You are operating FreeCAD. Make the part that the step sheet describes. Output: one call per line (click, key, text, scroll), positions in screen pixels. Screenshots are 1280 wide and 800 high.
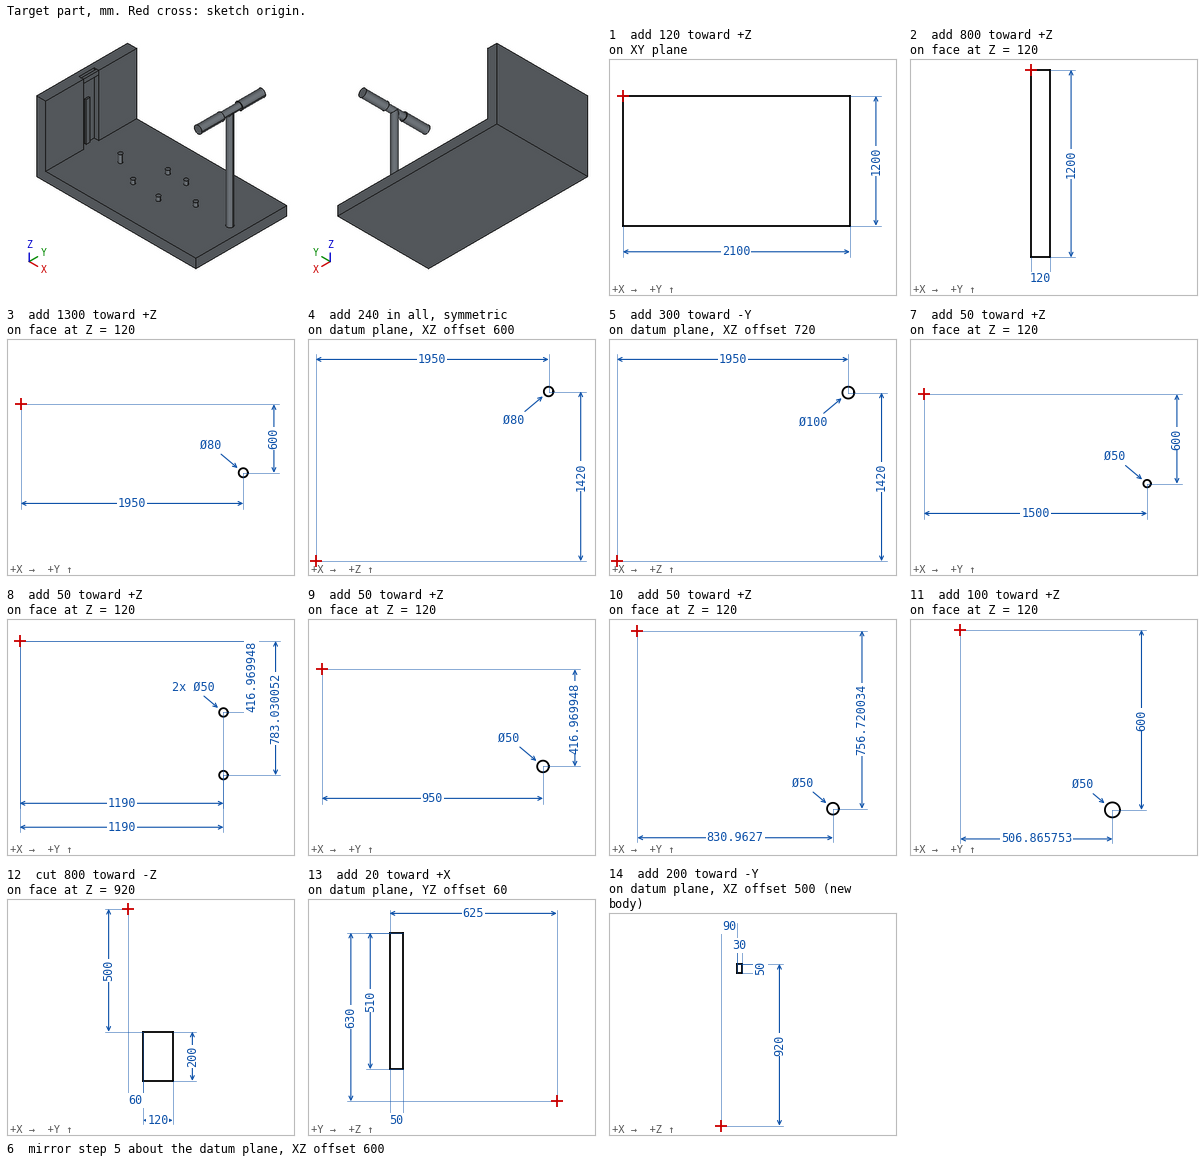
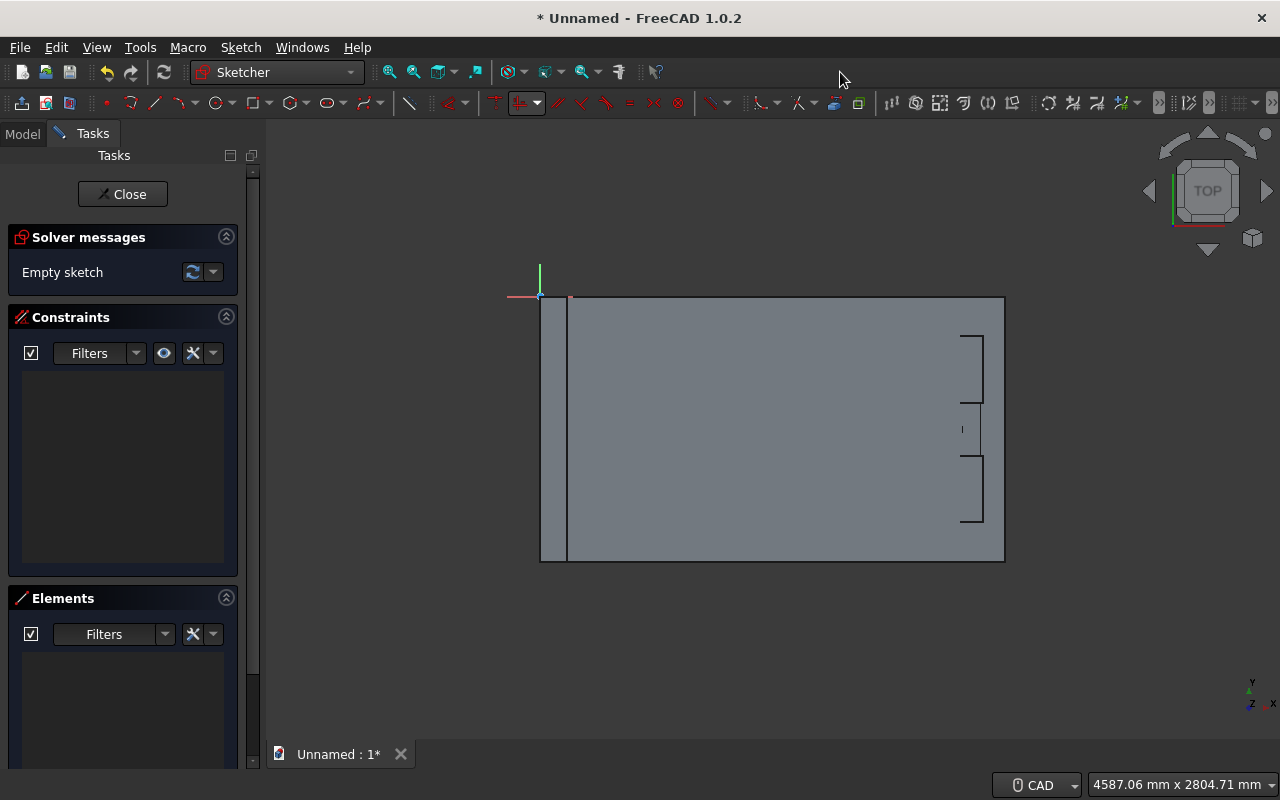
scroll(881, 429, up, 15)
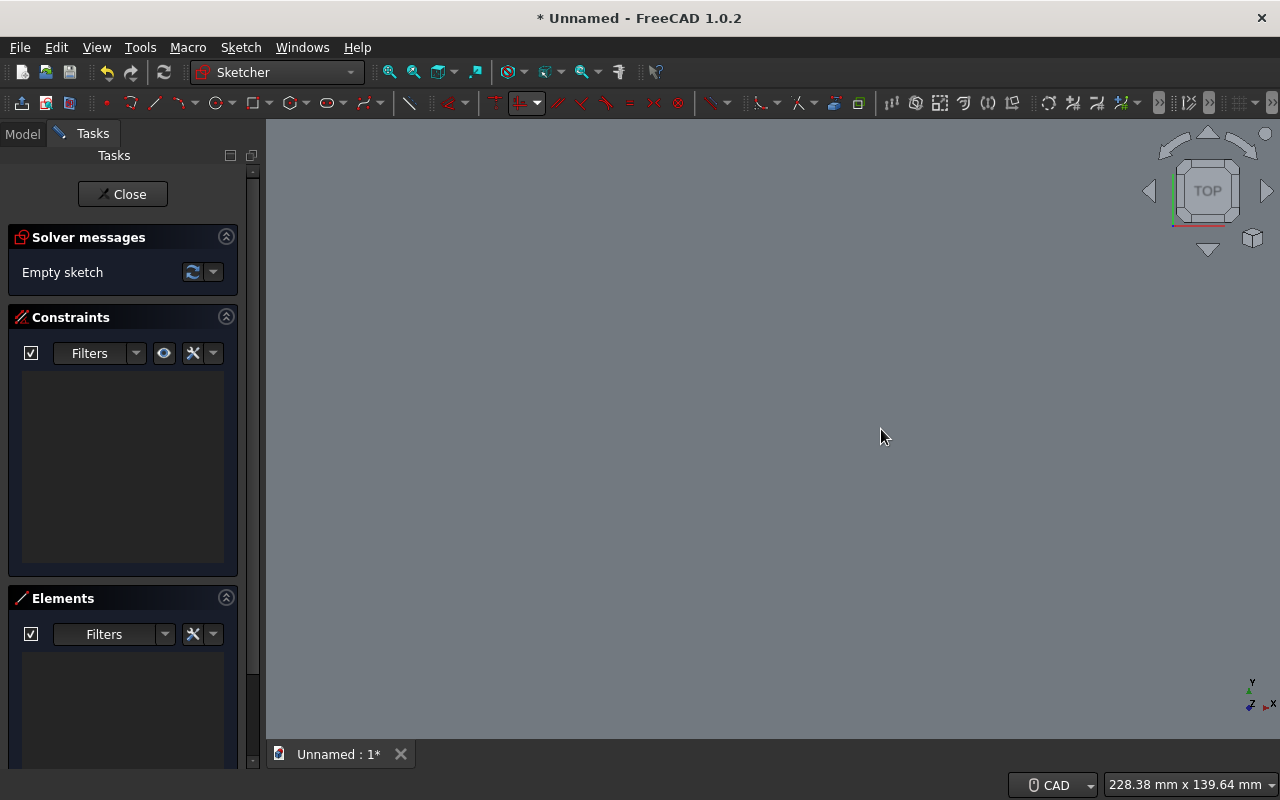
scroll(671, 416, up, 3)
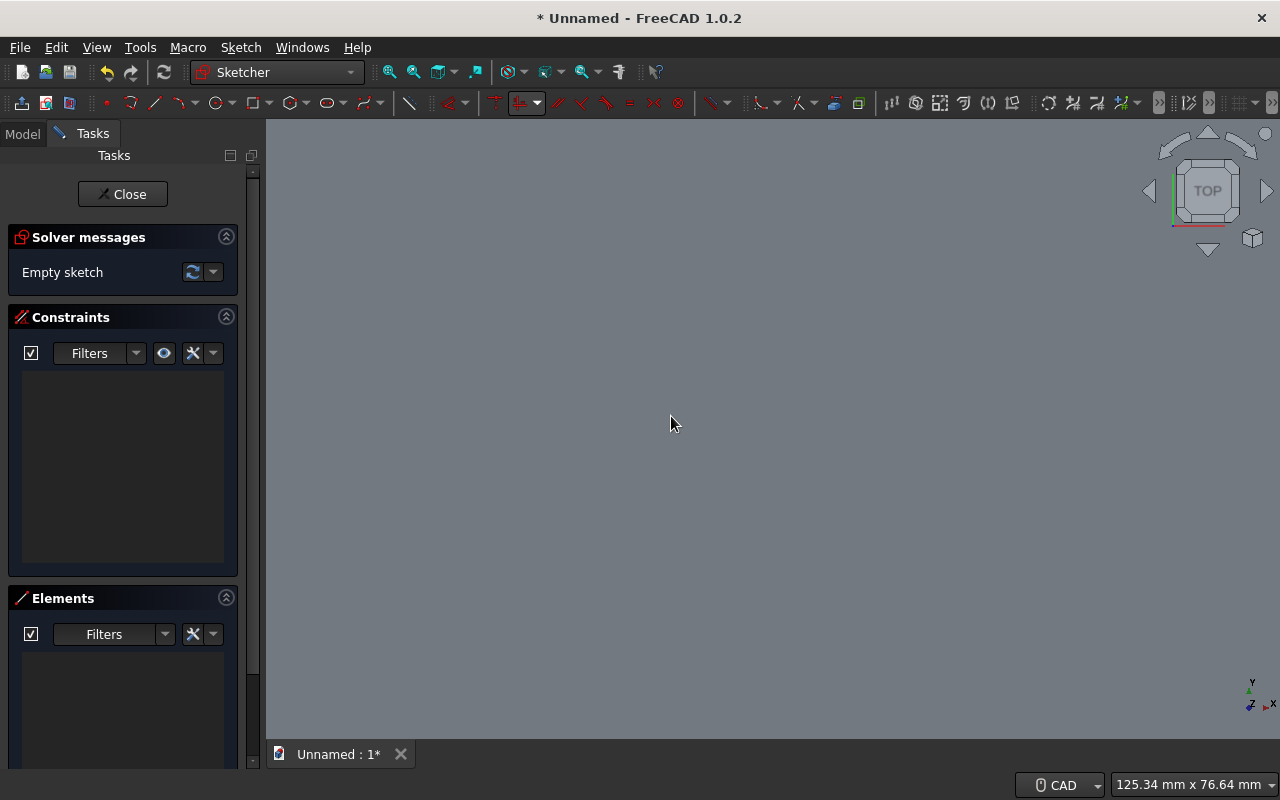
click(216, 104)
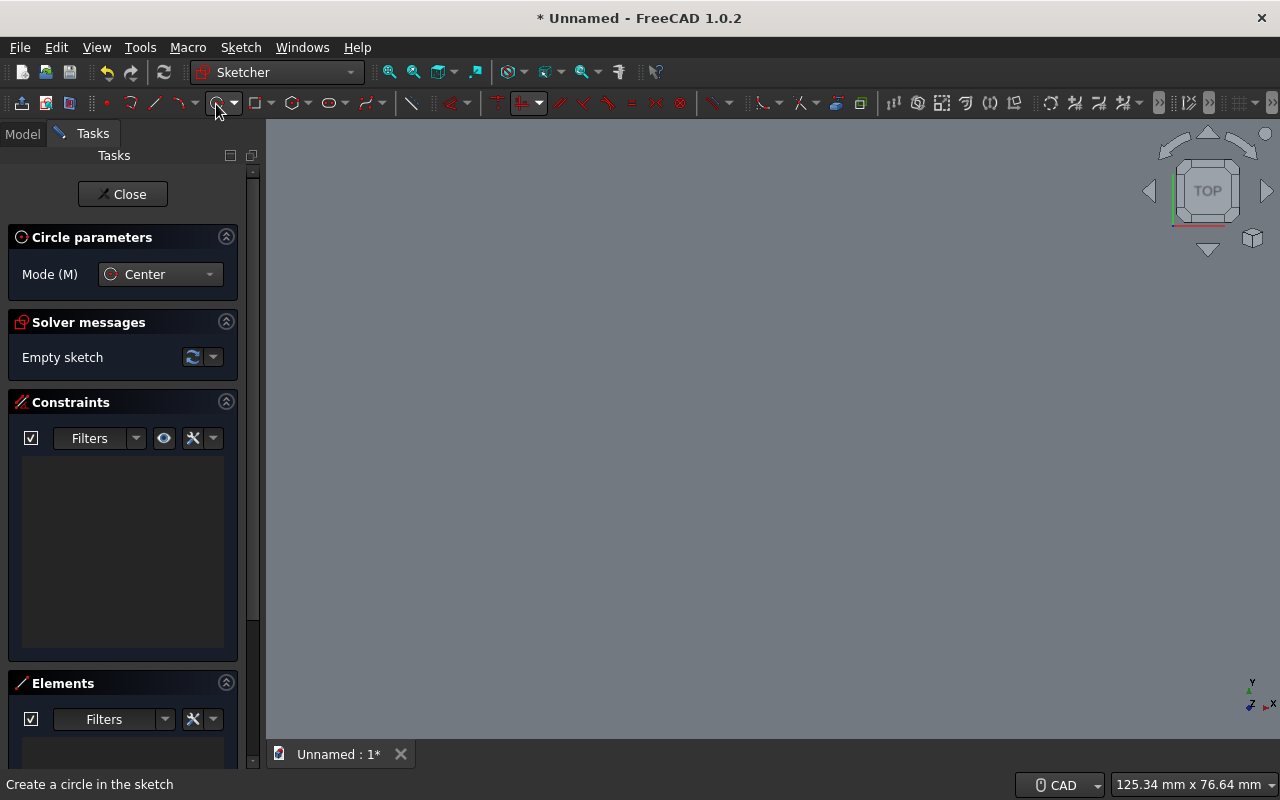
click(705, 429)
move(848, 285)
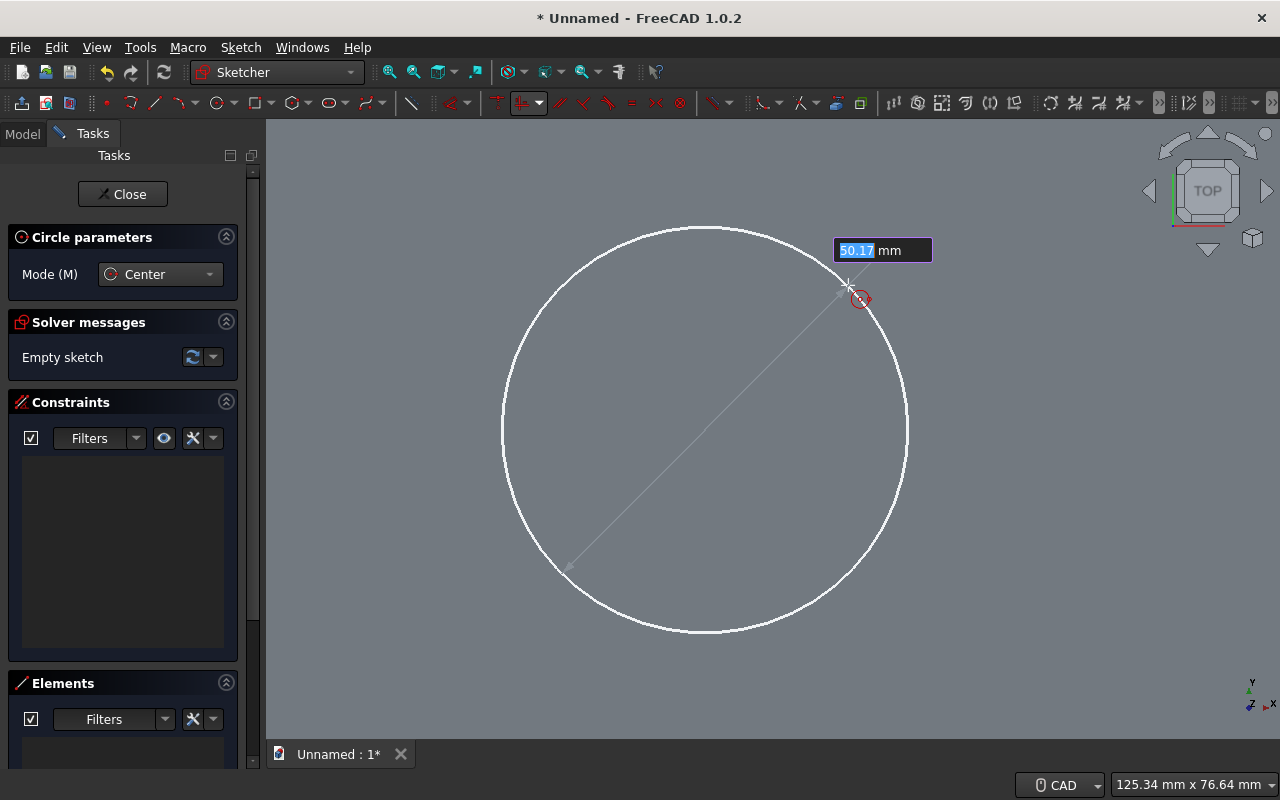
text(50)
key(Return)
key(Escape)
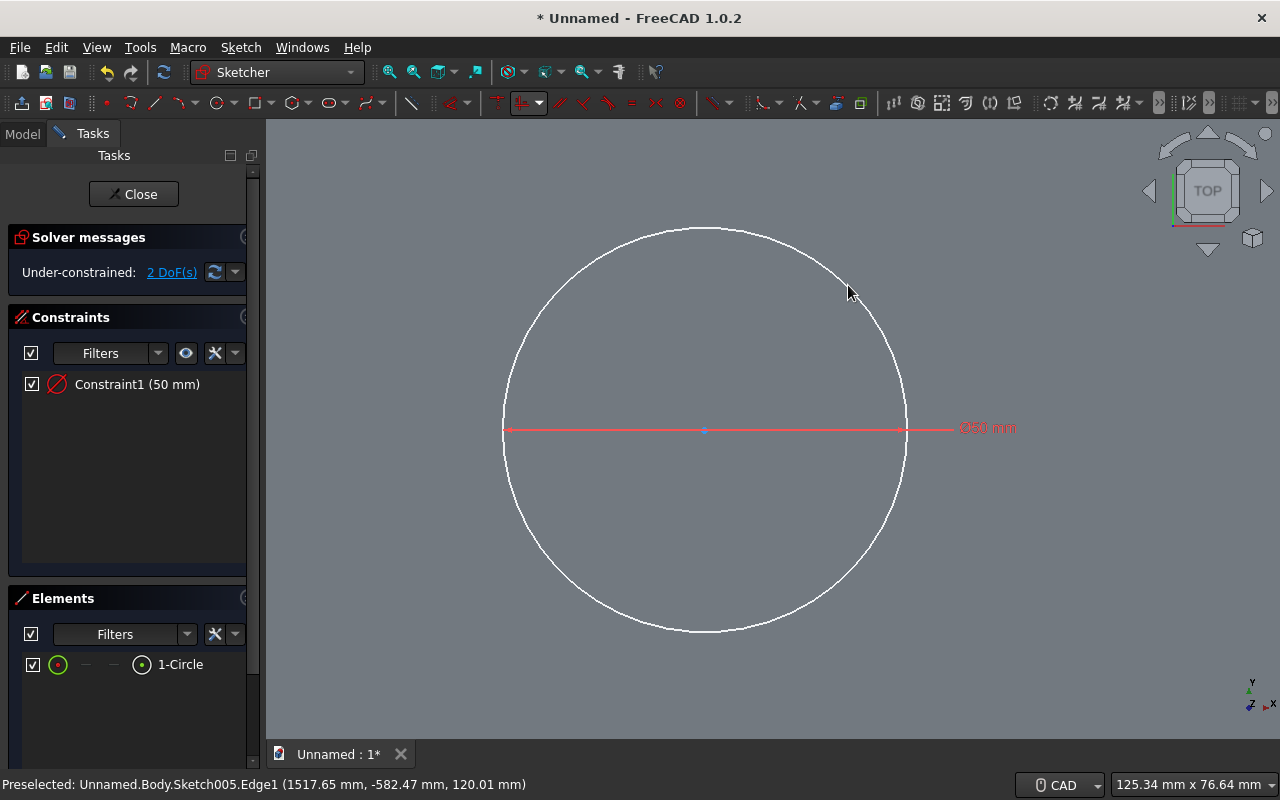
click(450, 104)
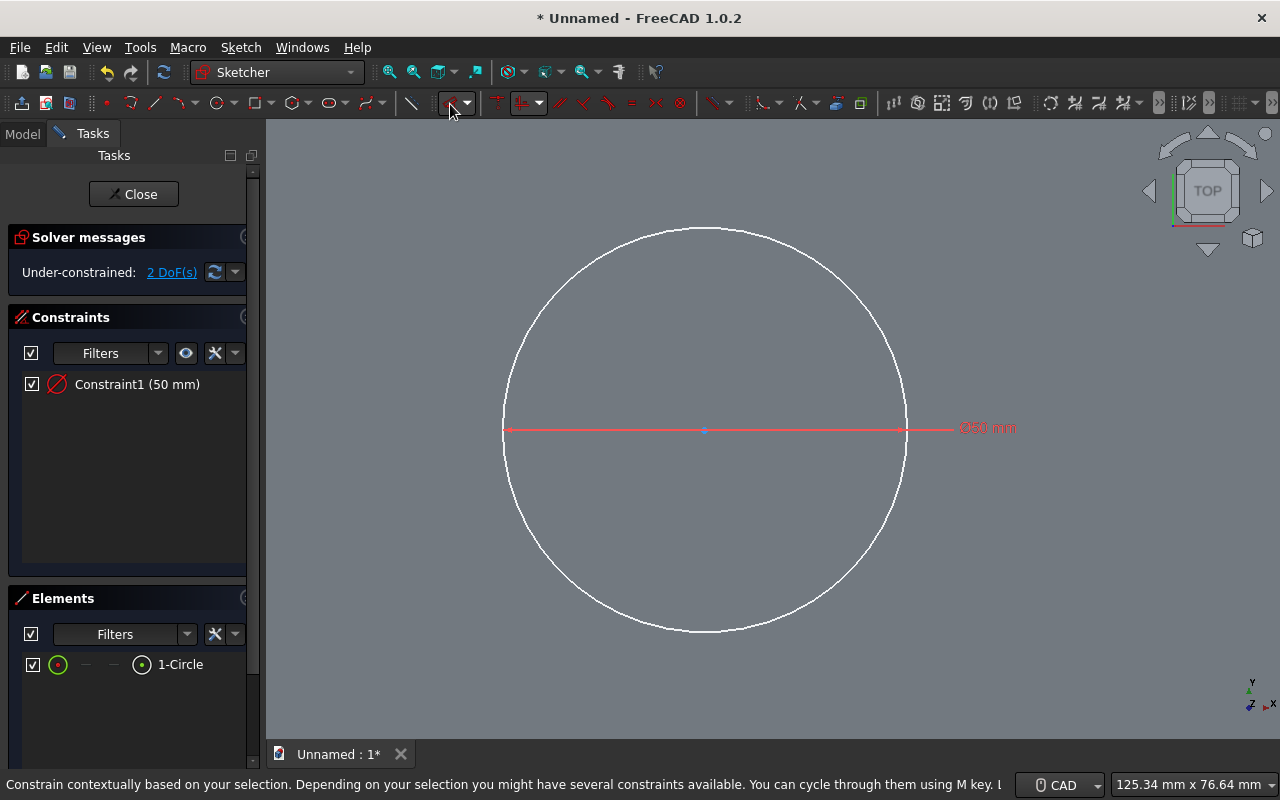
click(705, 430)
click(739, 288)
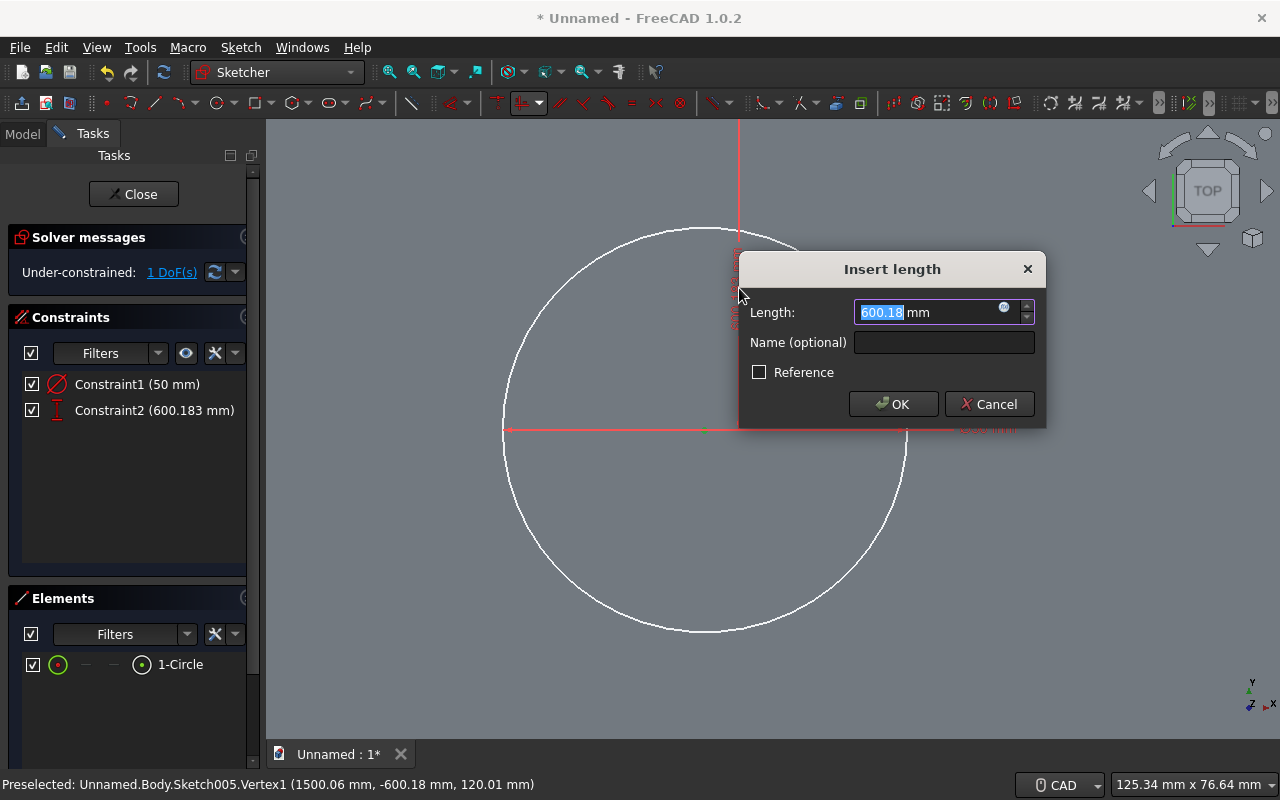
text(600)
key(Return)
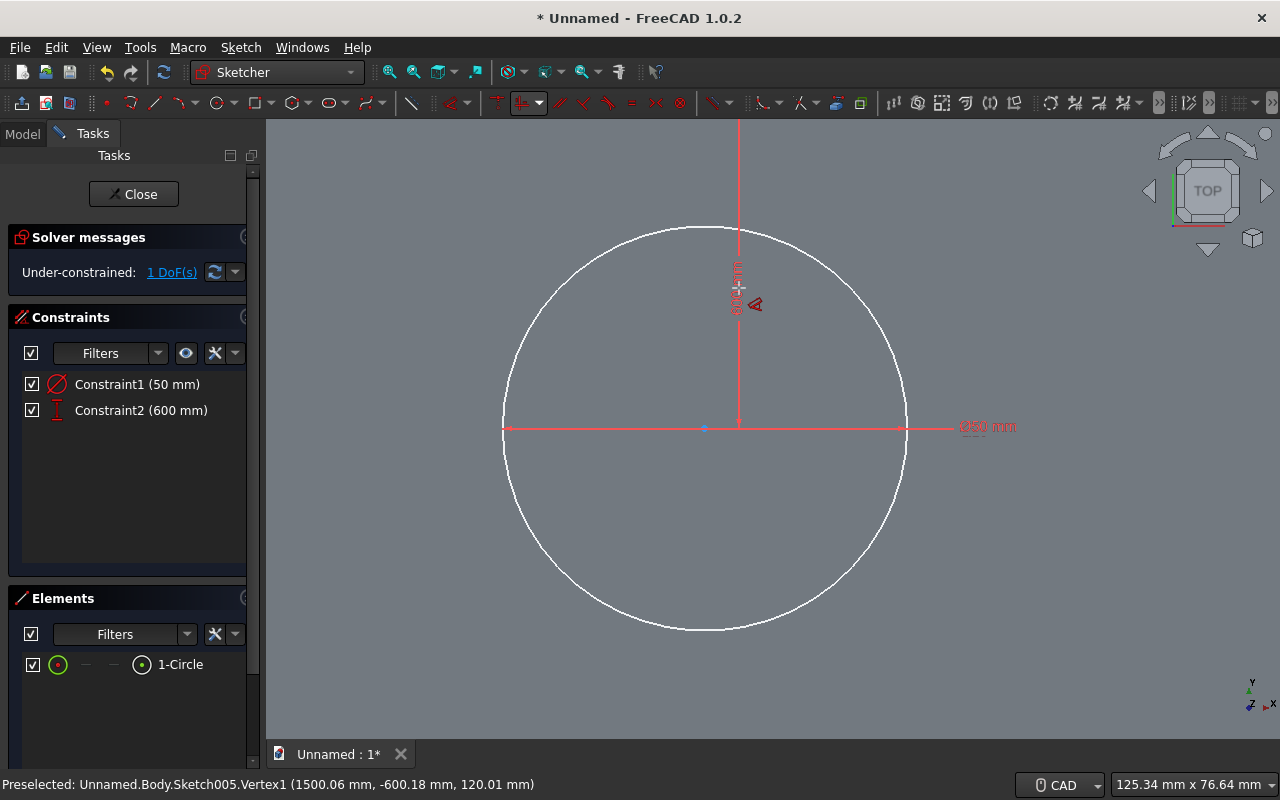
click(705, 429)
click(405, 463)